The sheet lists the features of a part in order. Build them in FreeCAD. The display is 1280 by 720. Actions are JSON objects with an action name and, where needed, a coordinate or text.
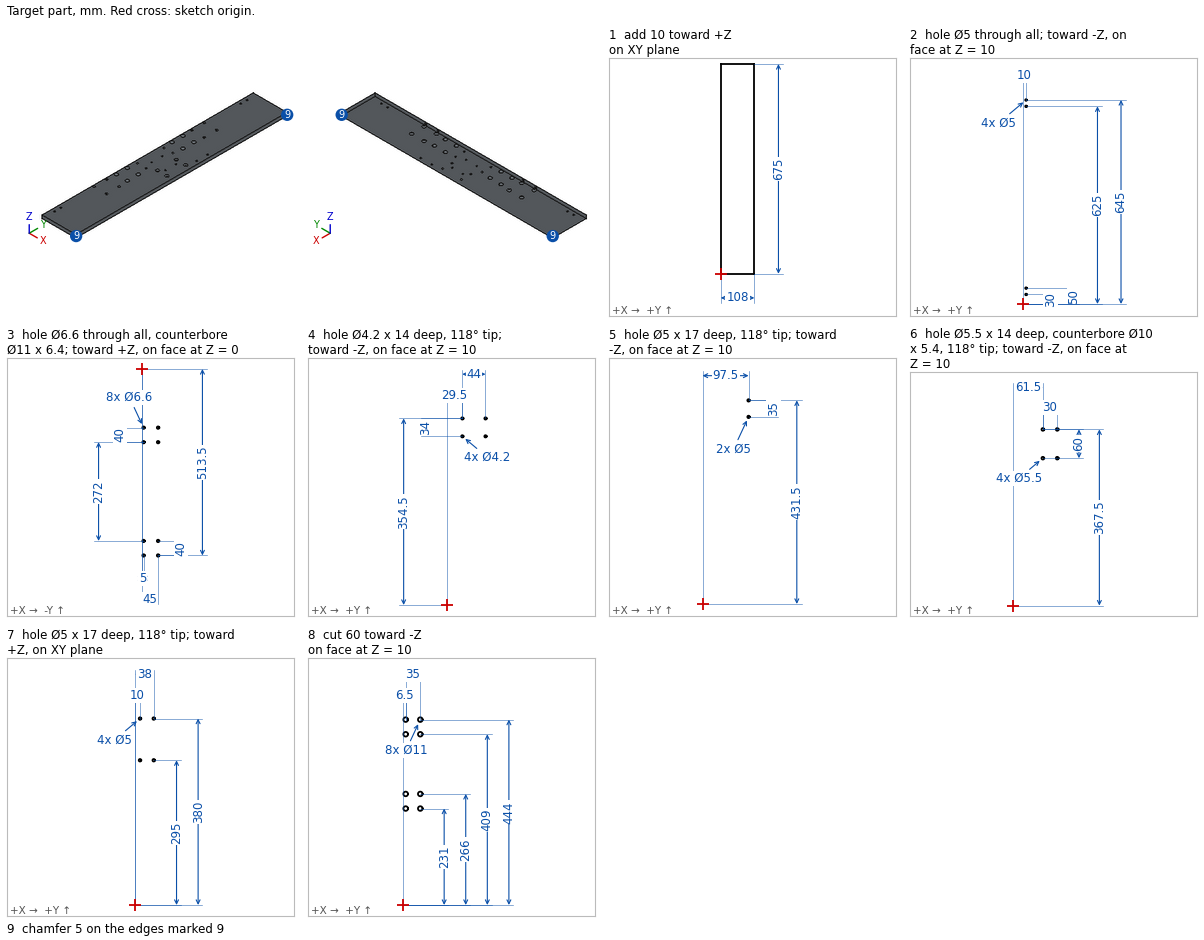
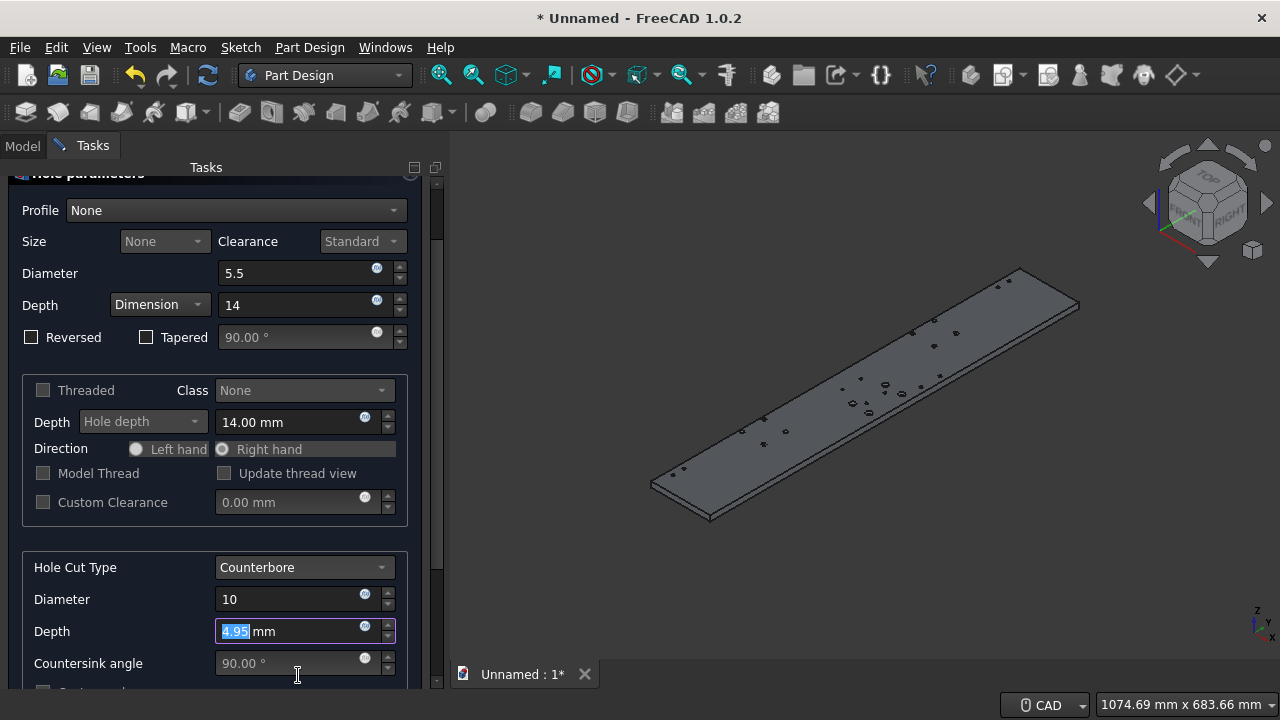
{"action": "type", "text": "5.4"}
{"action": "key", "text": "Tab"}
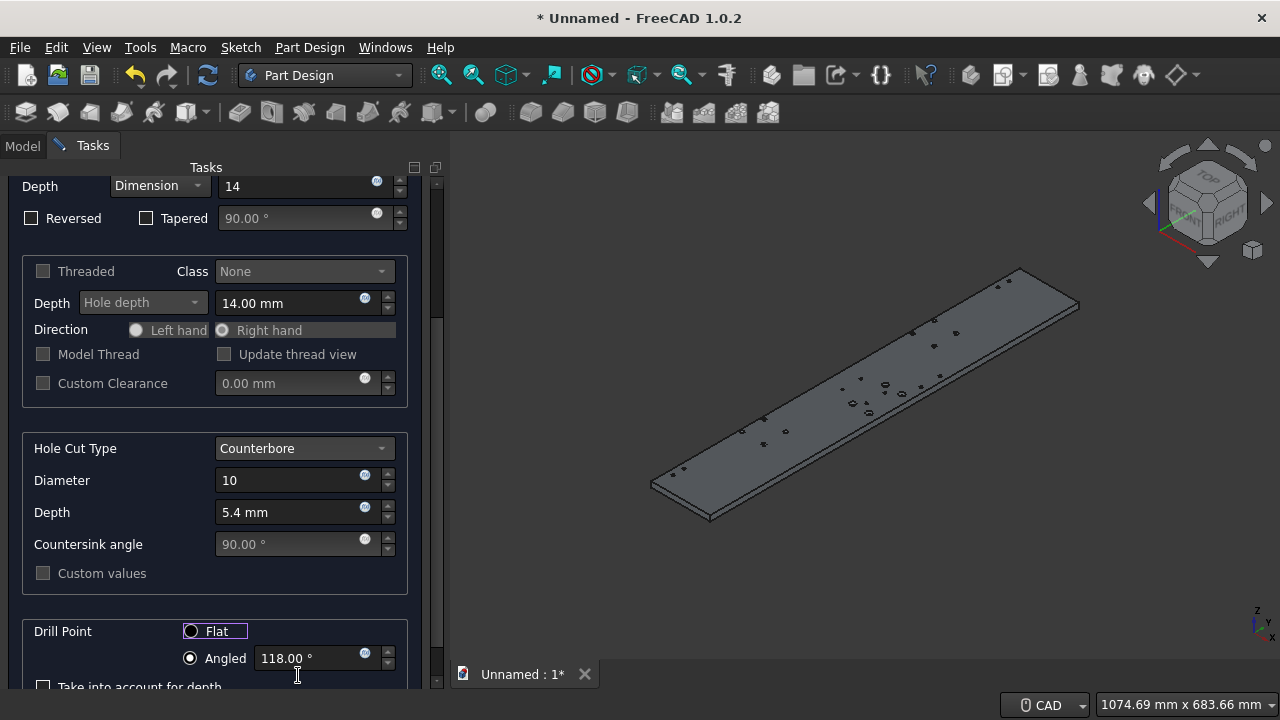
{"action": "scroll", "coordinate": [437, 432], "scroll_direction": "up", "scroll_amount": 4}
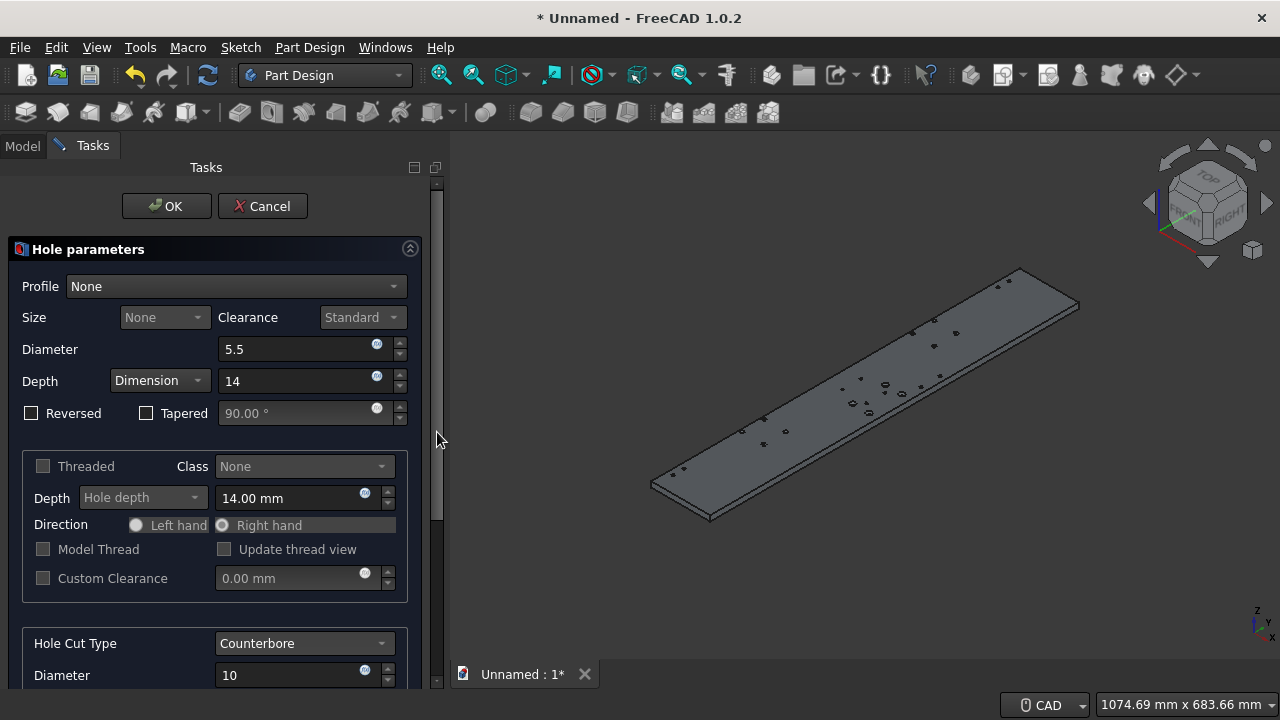
{"action": "left_click", "coordinate": [167, 206]}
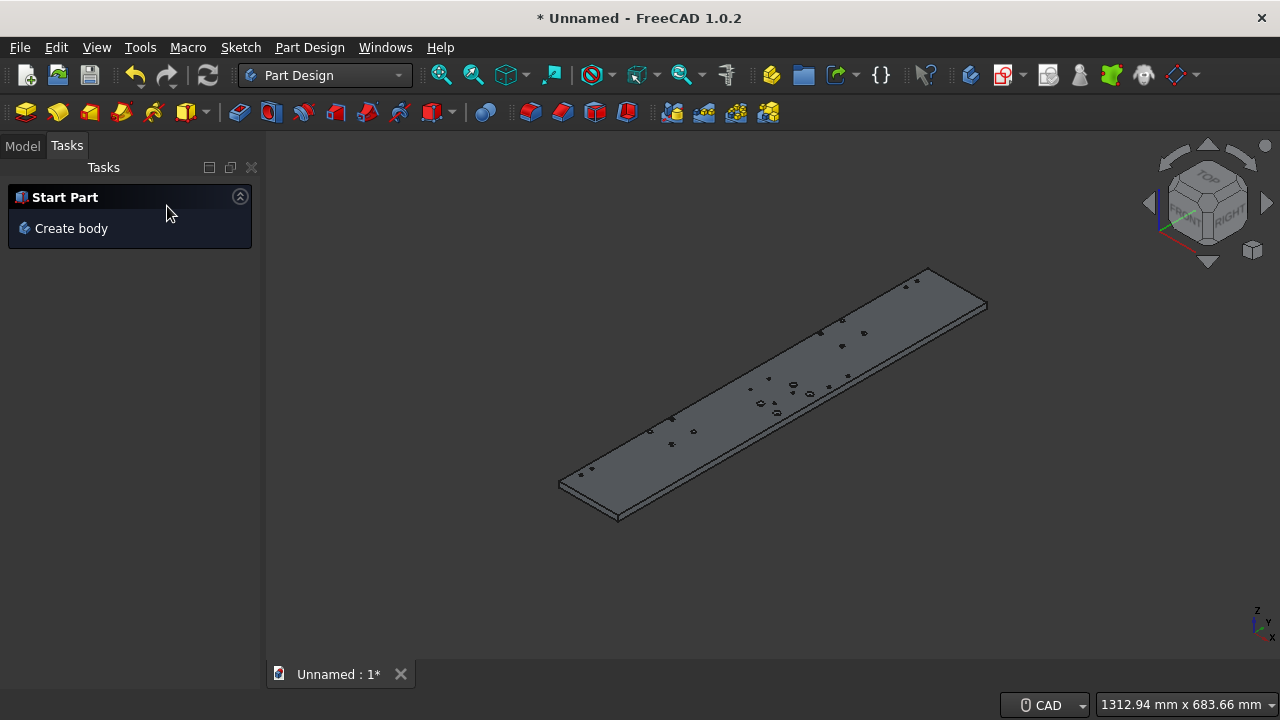
{"action": "left_click", "coordinate": [1004, 76]}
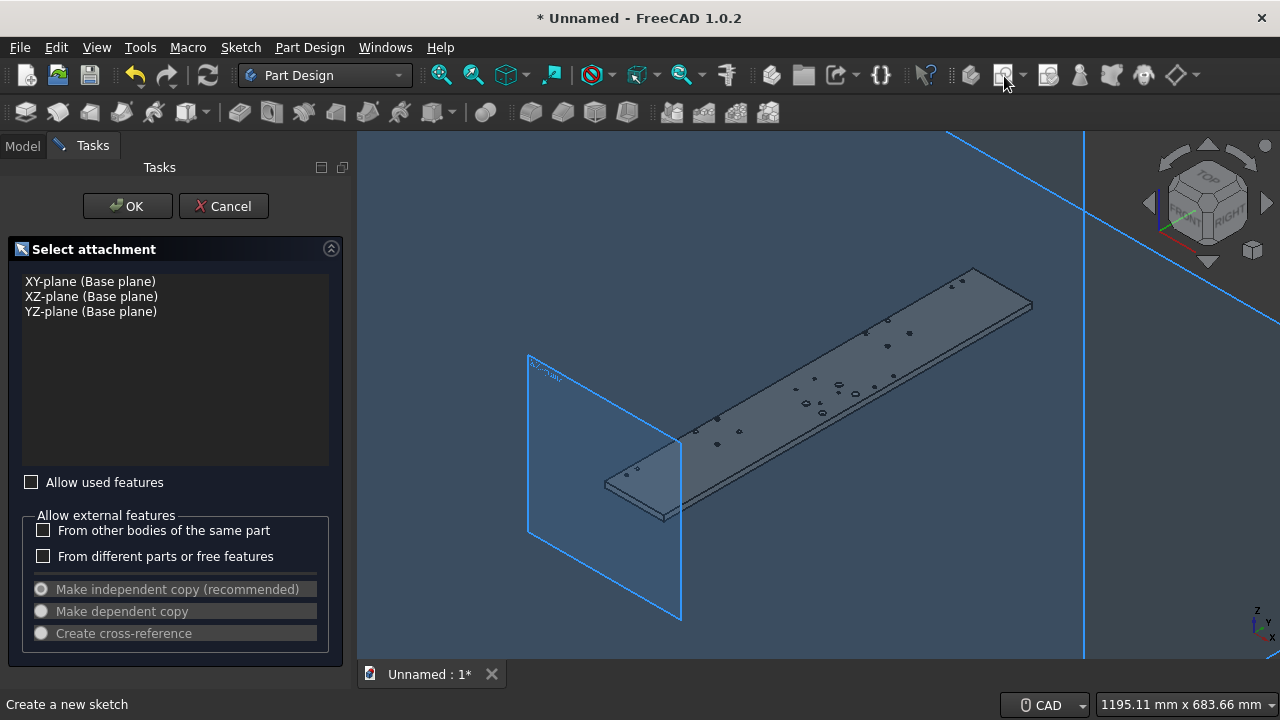
{"action": "left_click", "coordinate": [82, 282]}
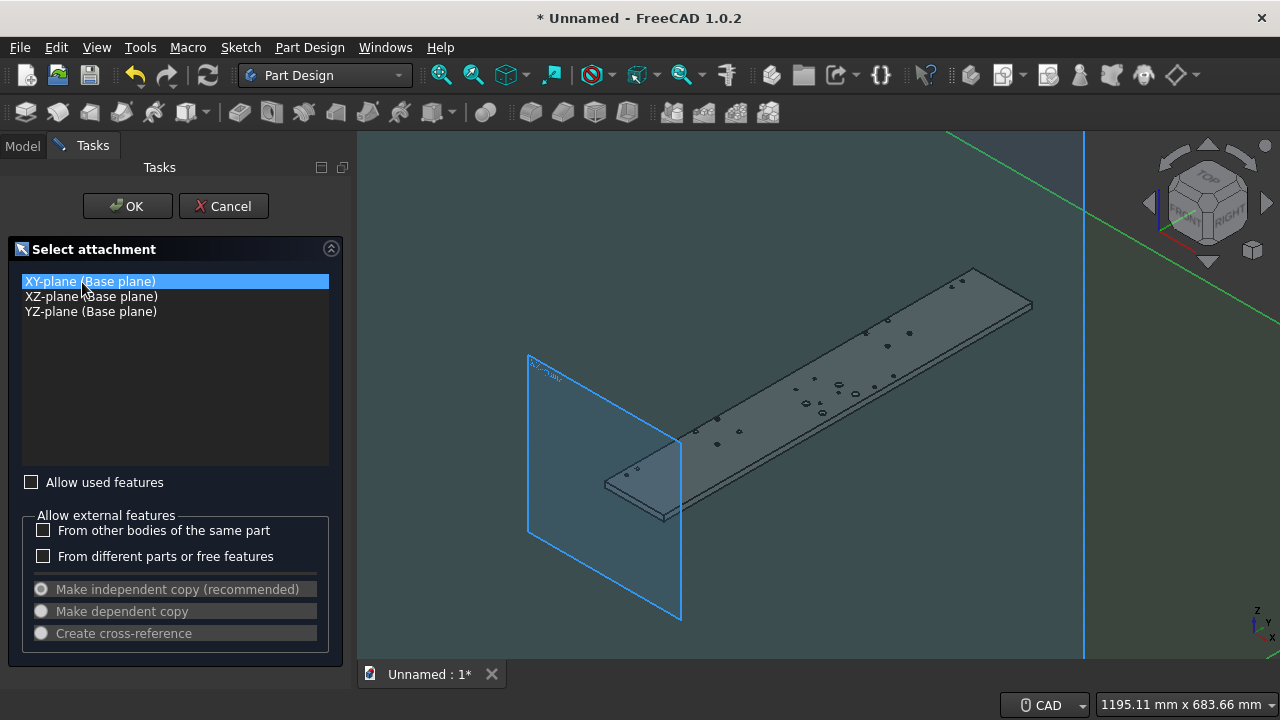
{"action": "left_click", "coordinate": [128, 206]}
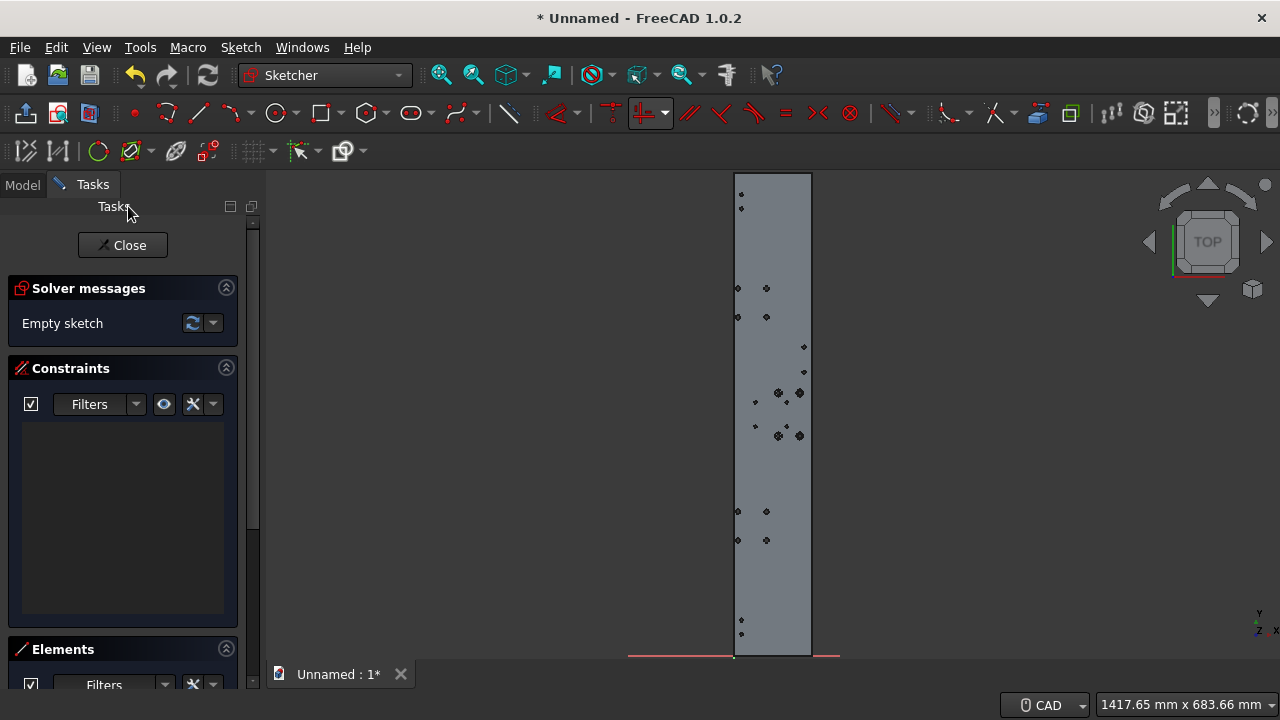
{"action": "left_click", "coordinate": [90, 114]}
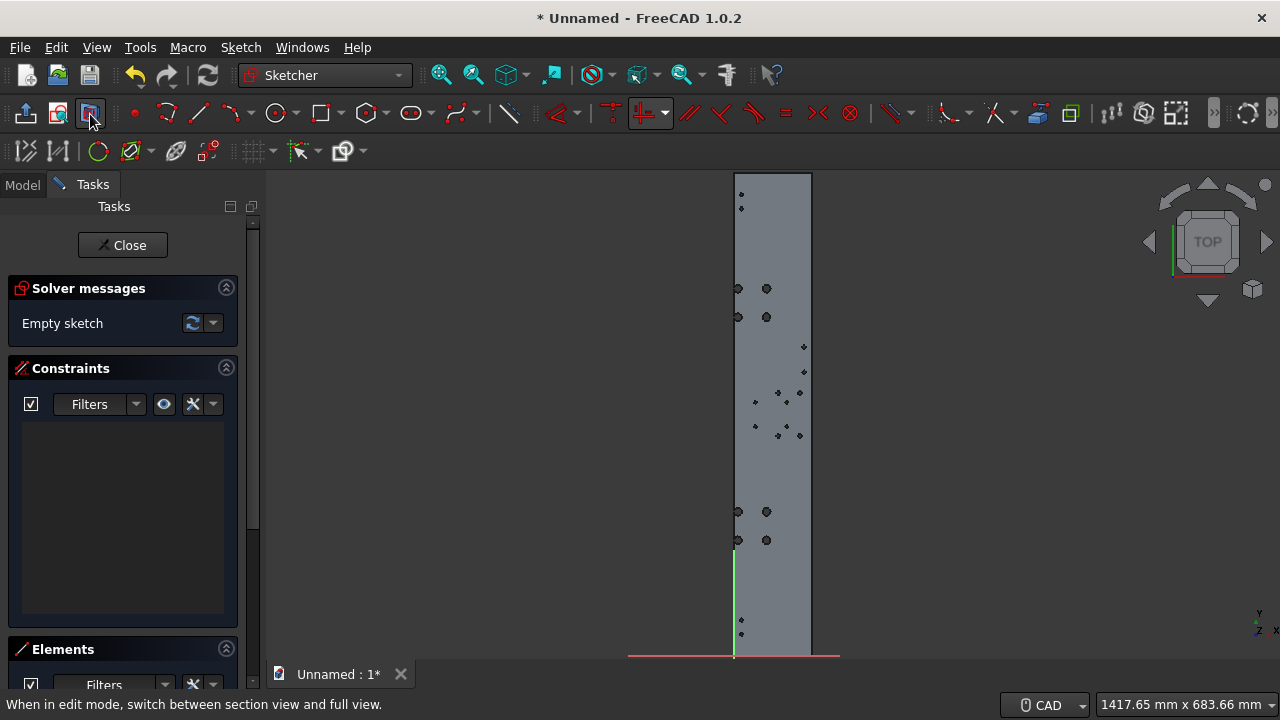
{"action": "scroll", "coordinate": [763, 414], "scroll_direction": "up", "scroll_amount": 8}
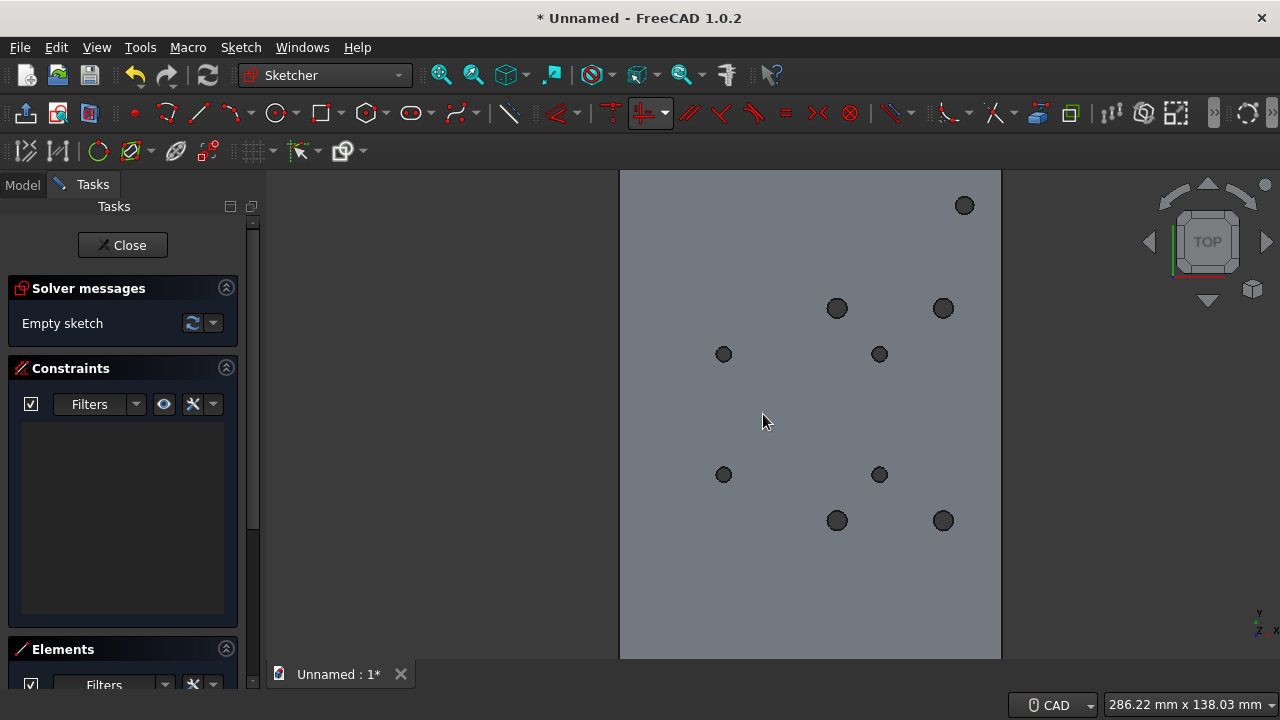
{"action": "left_click", "coordinate": [276, 114]}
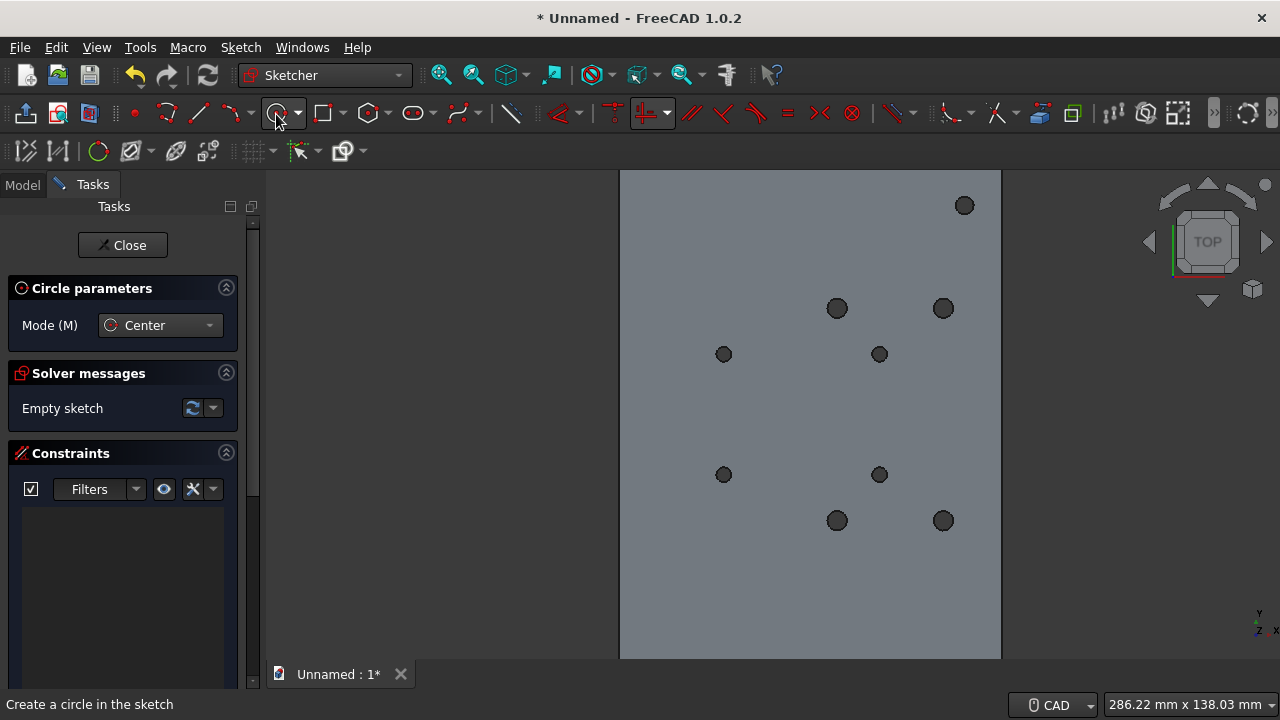
{"action": "scroll", "coordinate": [754, 264], "scroll_direction": "up", "scroll_amount": 5}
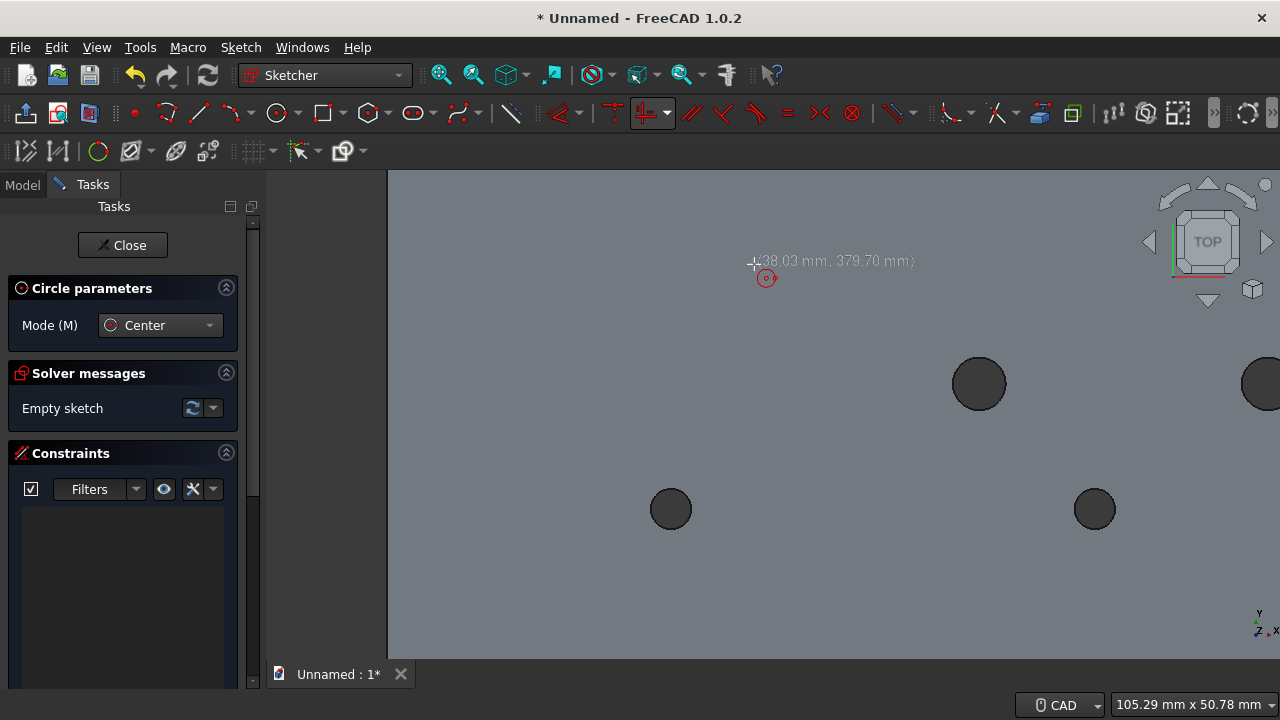
{"action": "left_click", "coordinate": [753, 263]}
{"action": "mouse_move", "coordinate": [770, 246]}